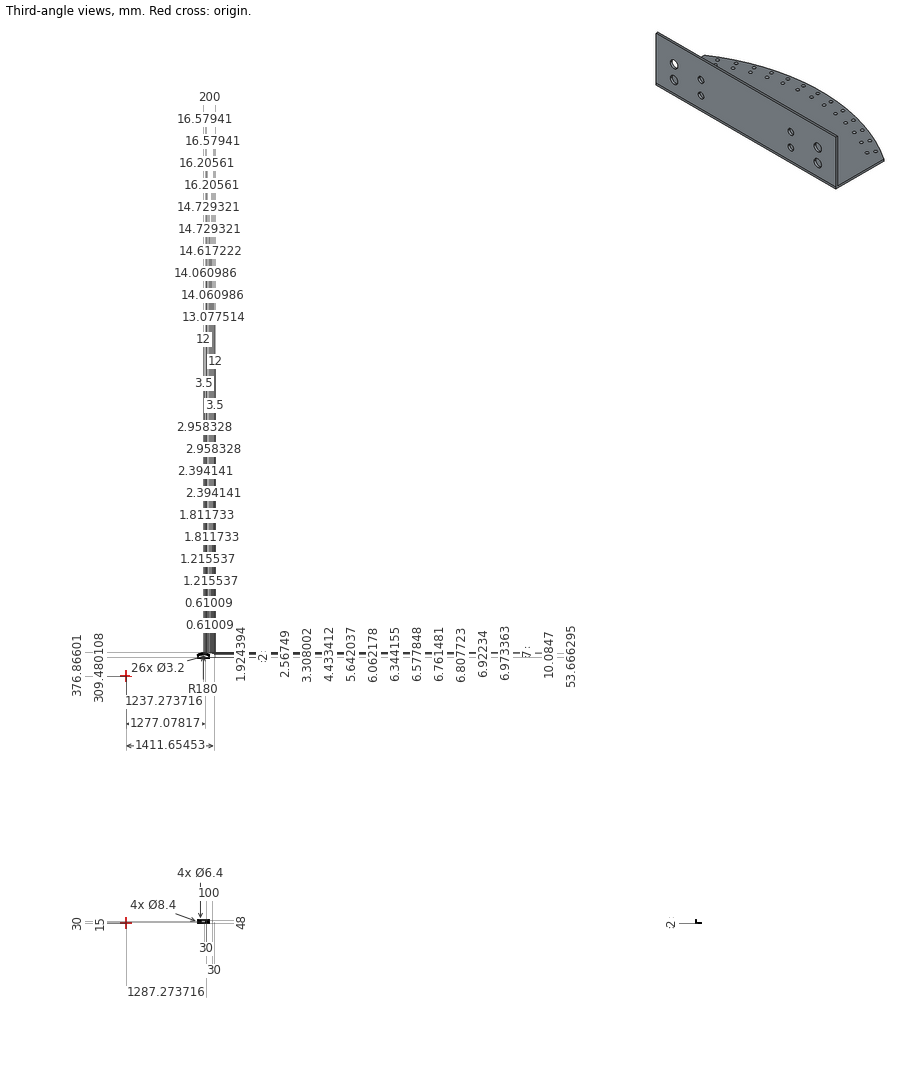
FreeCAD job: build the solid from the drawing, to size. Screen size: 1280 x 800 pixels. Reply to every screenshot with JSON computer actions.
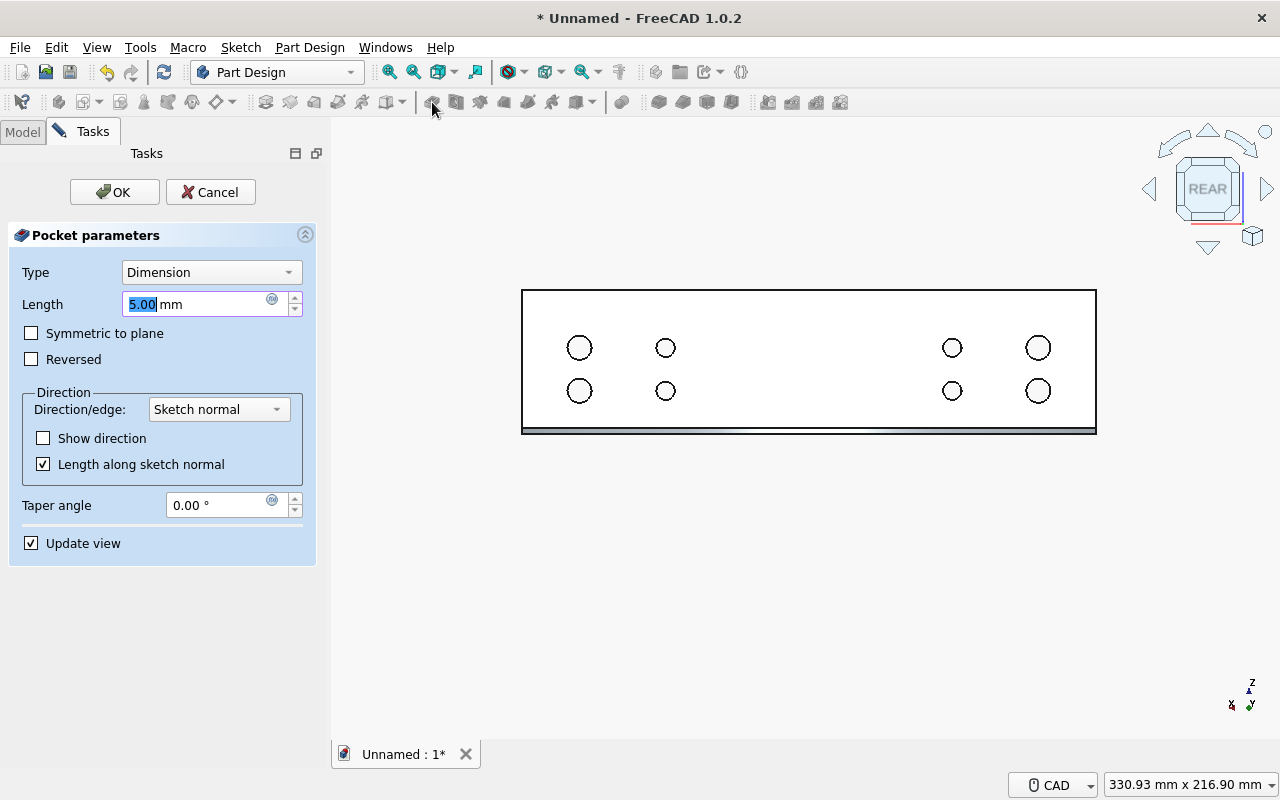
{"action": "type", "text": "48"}
{"action": "key", "text": "Tab"}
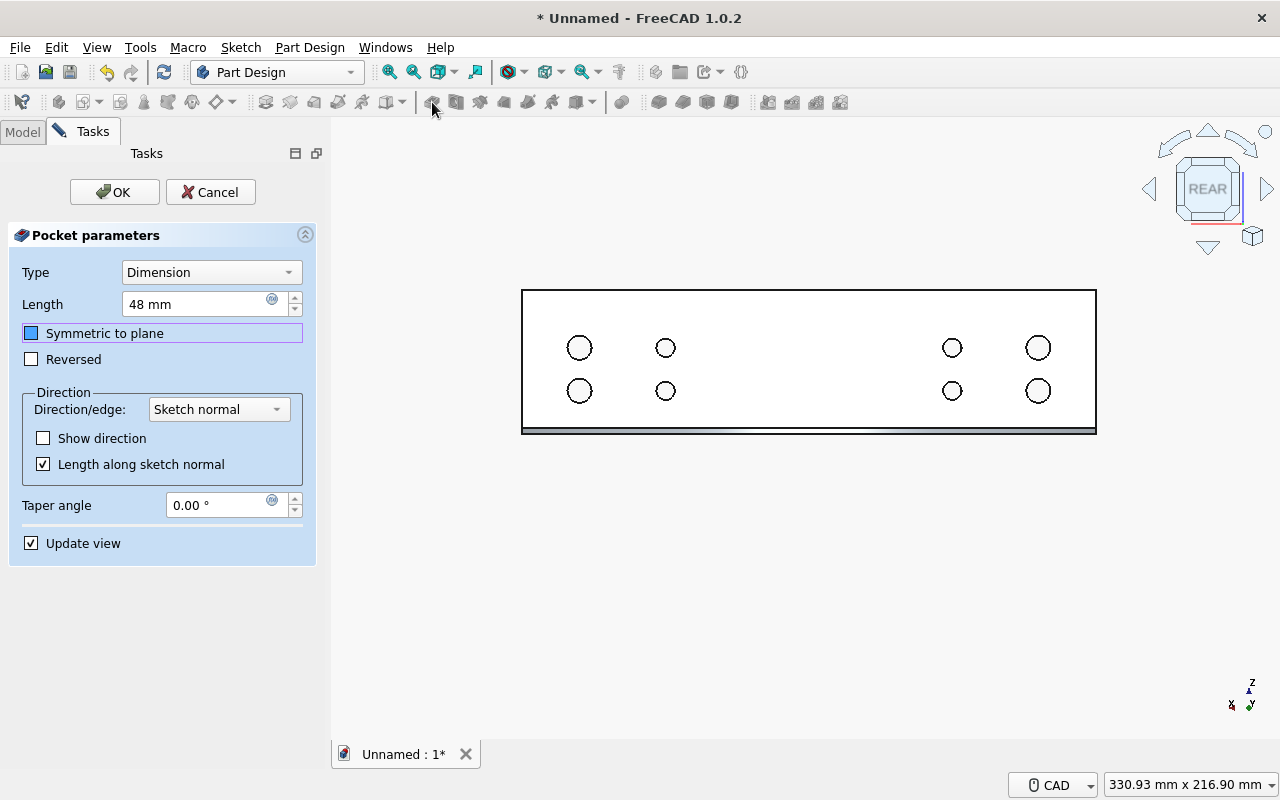
{"action": "left_click", "coordinate": [115, 192]}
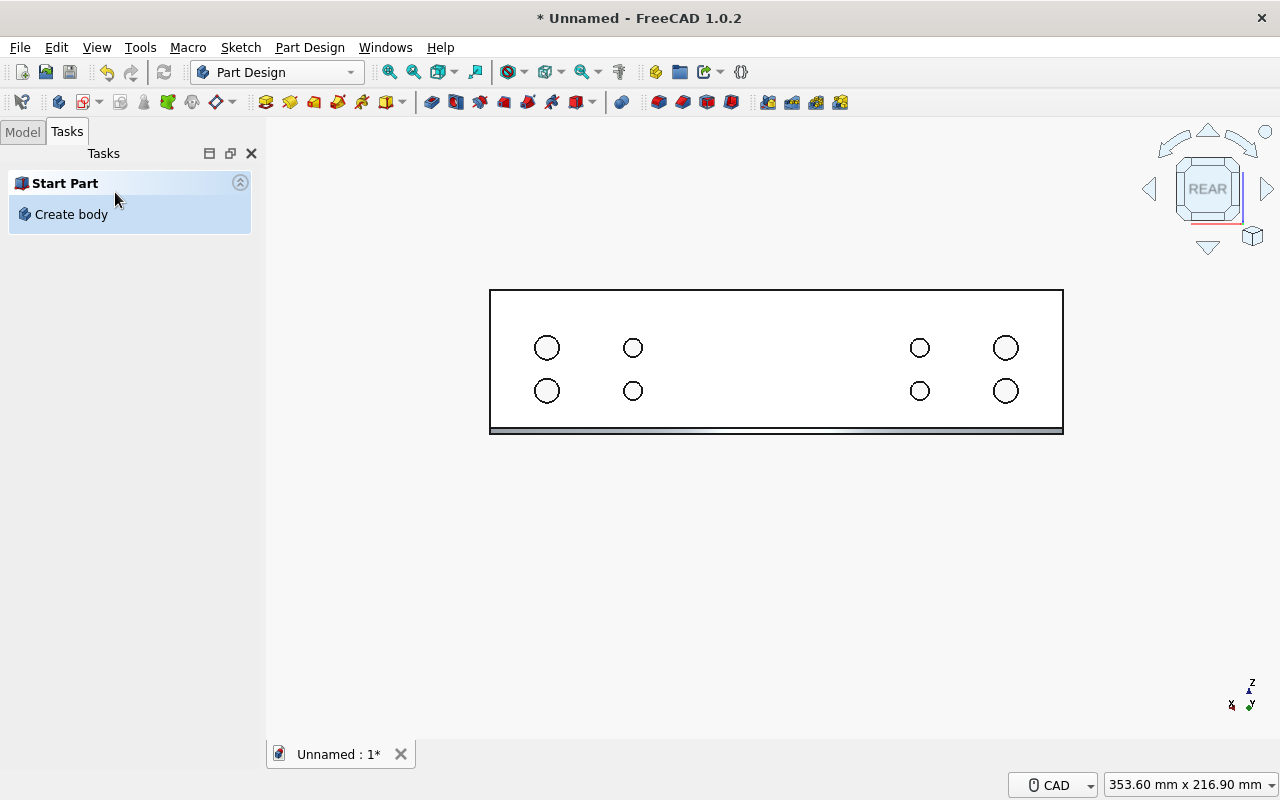
{"action": "key", "text": "0"}